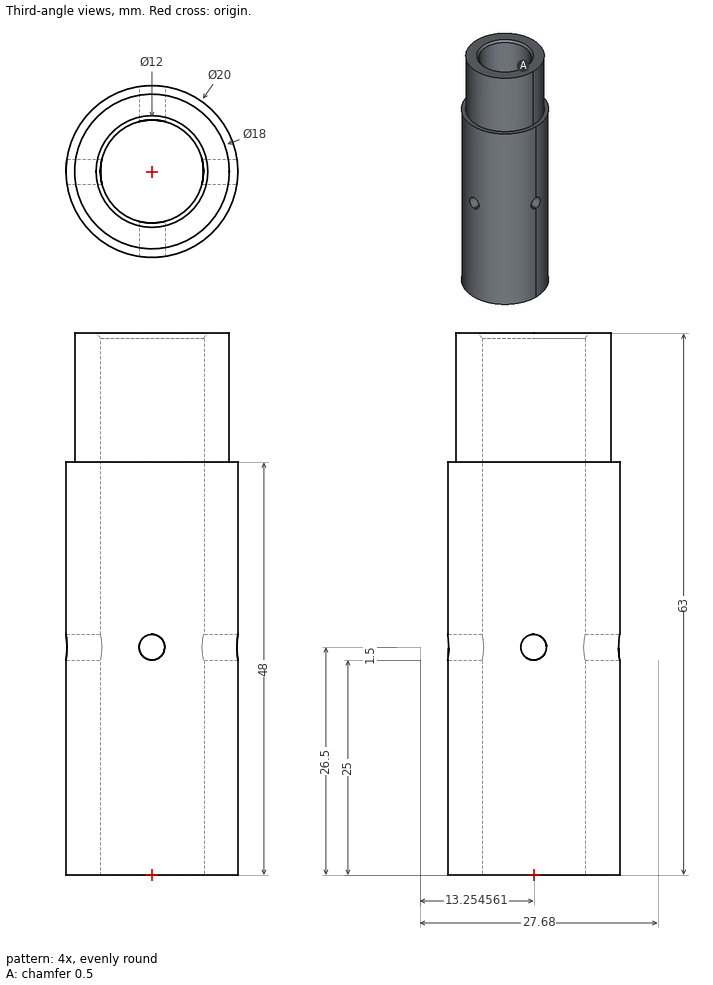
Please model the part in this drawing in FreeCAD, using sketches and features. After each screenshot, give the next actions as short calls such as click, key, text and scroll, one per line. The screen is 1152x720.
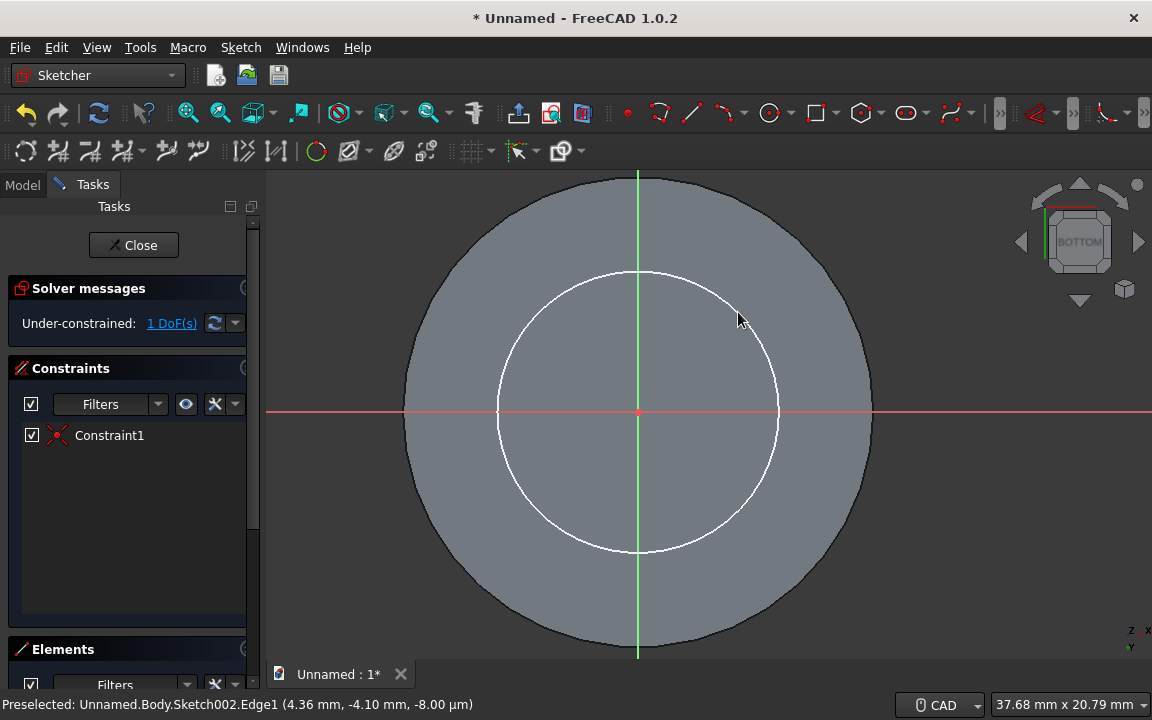
click(1036, 114)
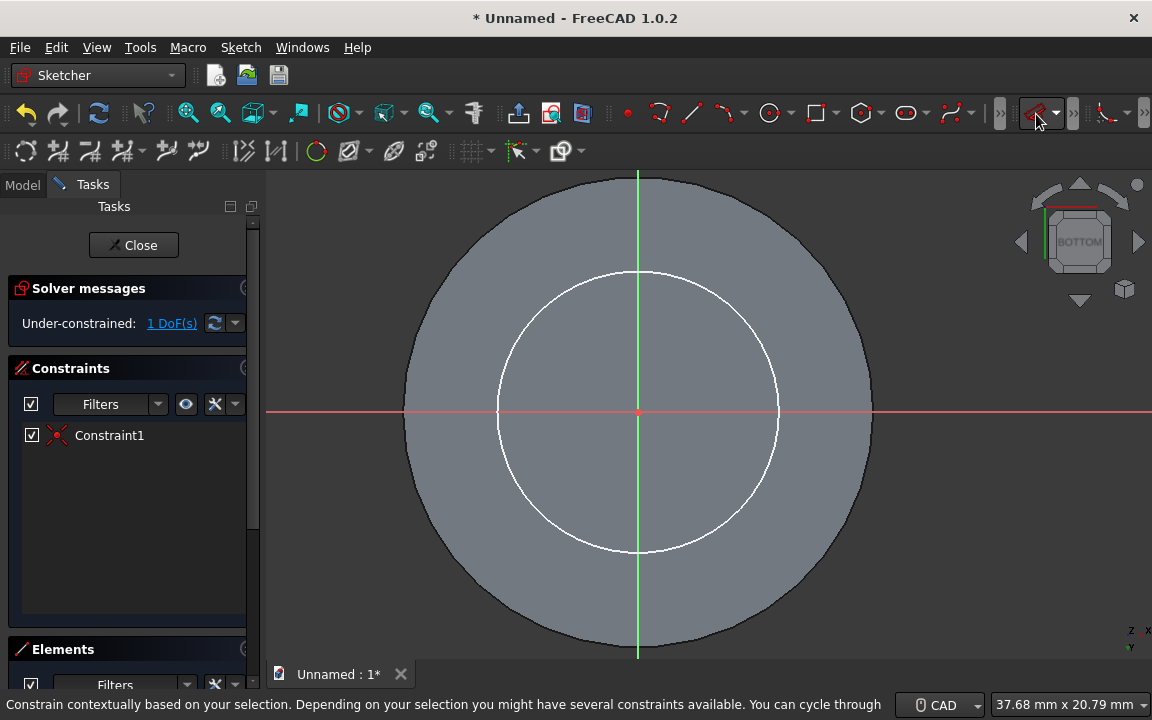
click(737, 312)
click(759, 289)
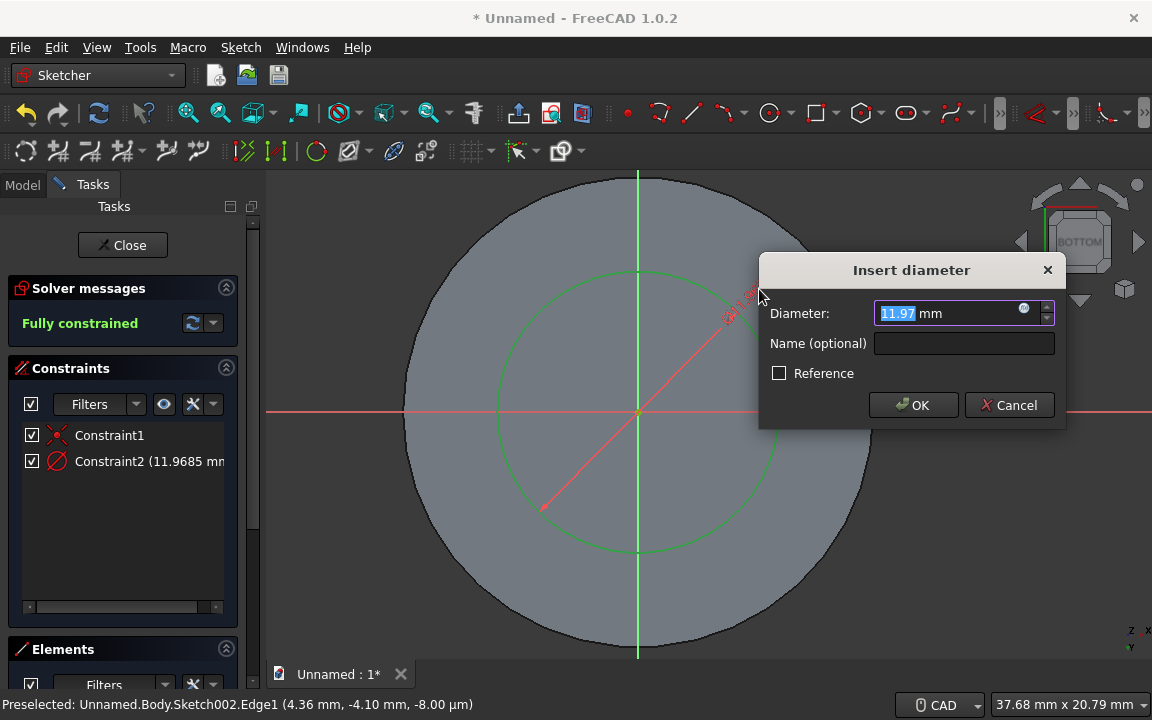
text(12)
key(Return)
key(Escape)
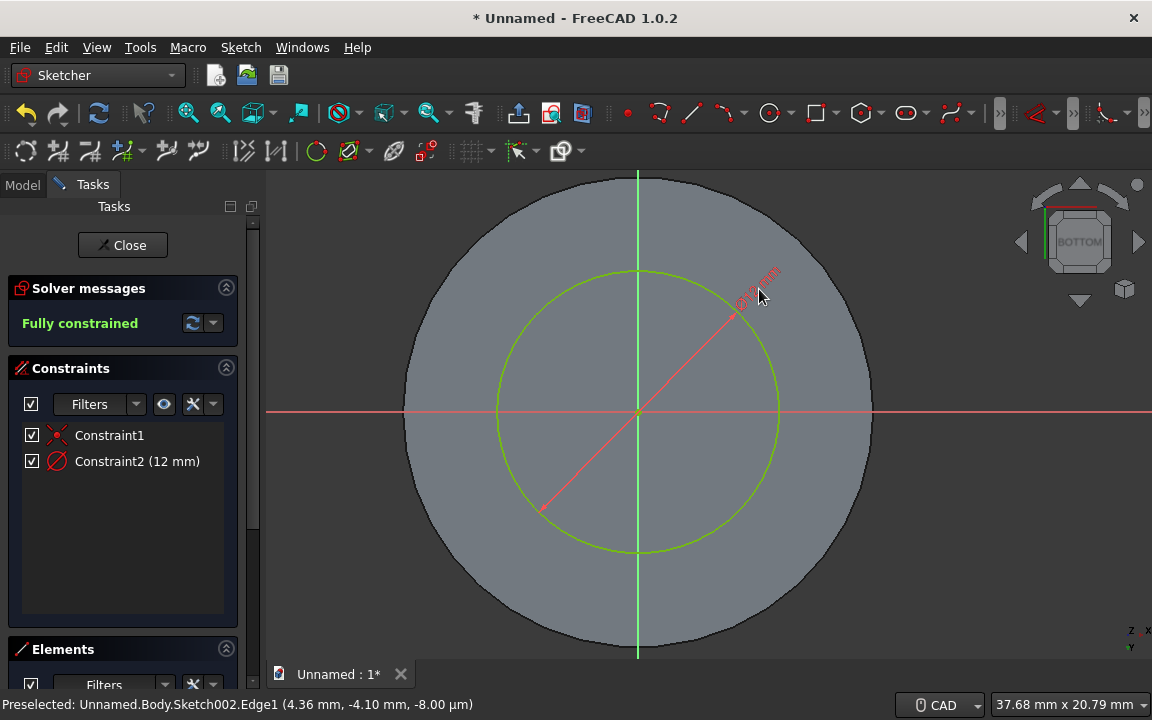
click(123, 245)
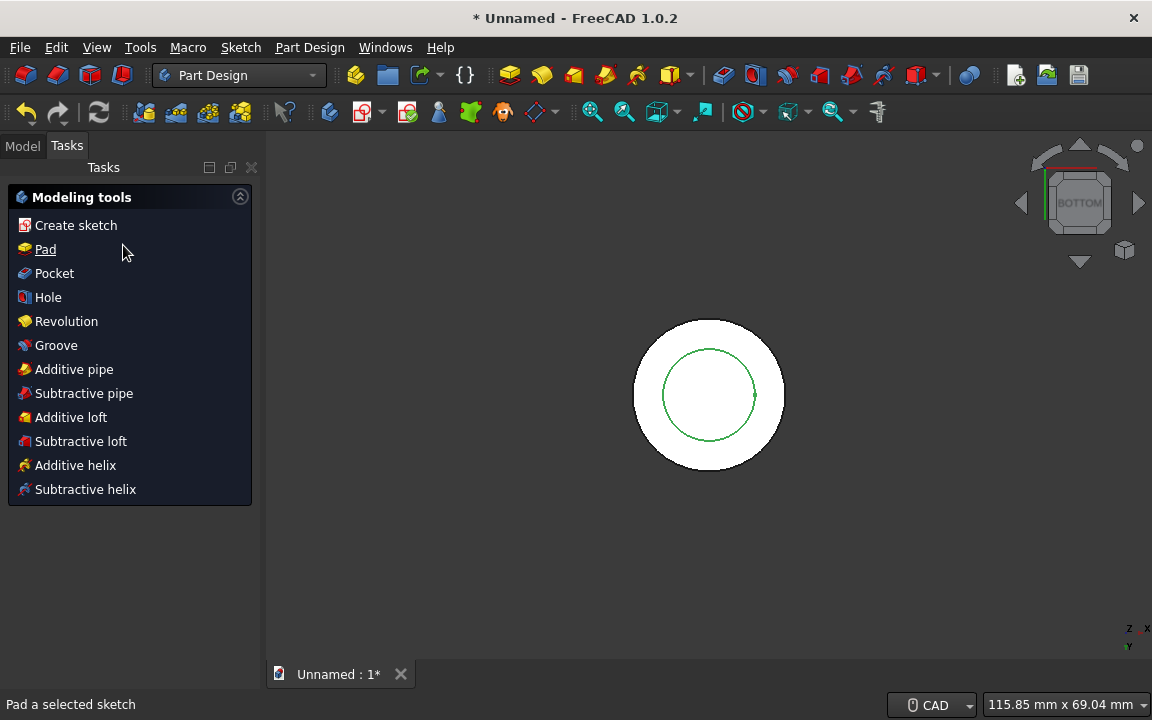
click(724, 76)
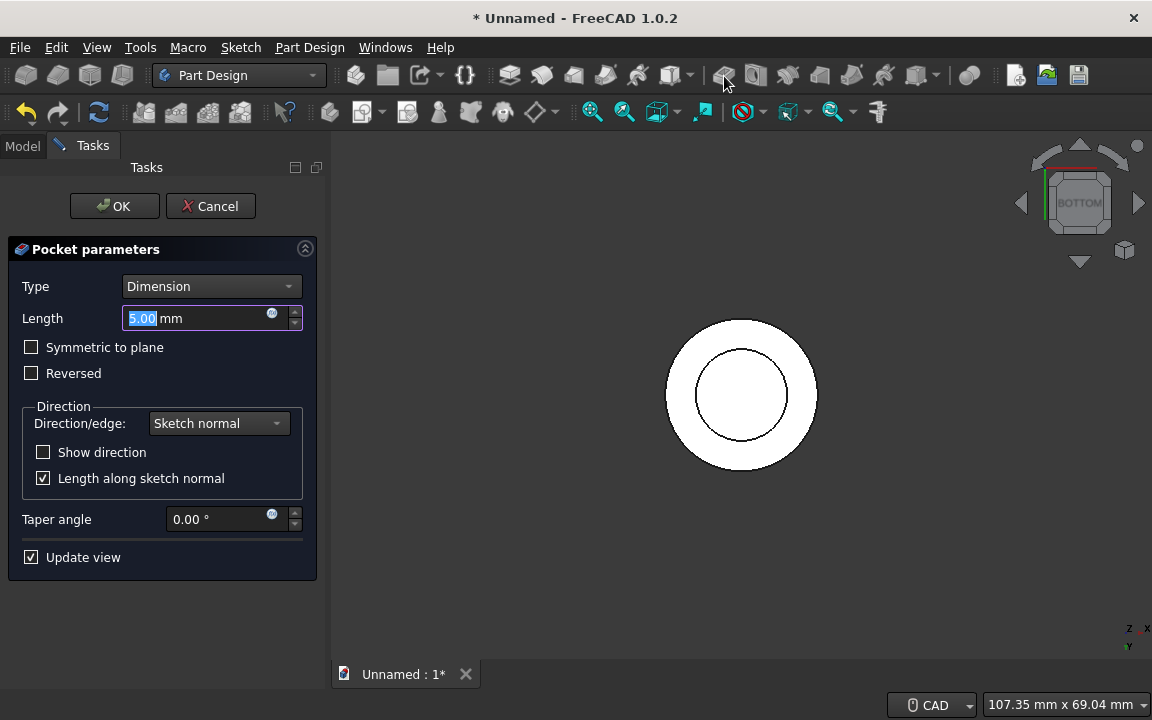
click(212, 286)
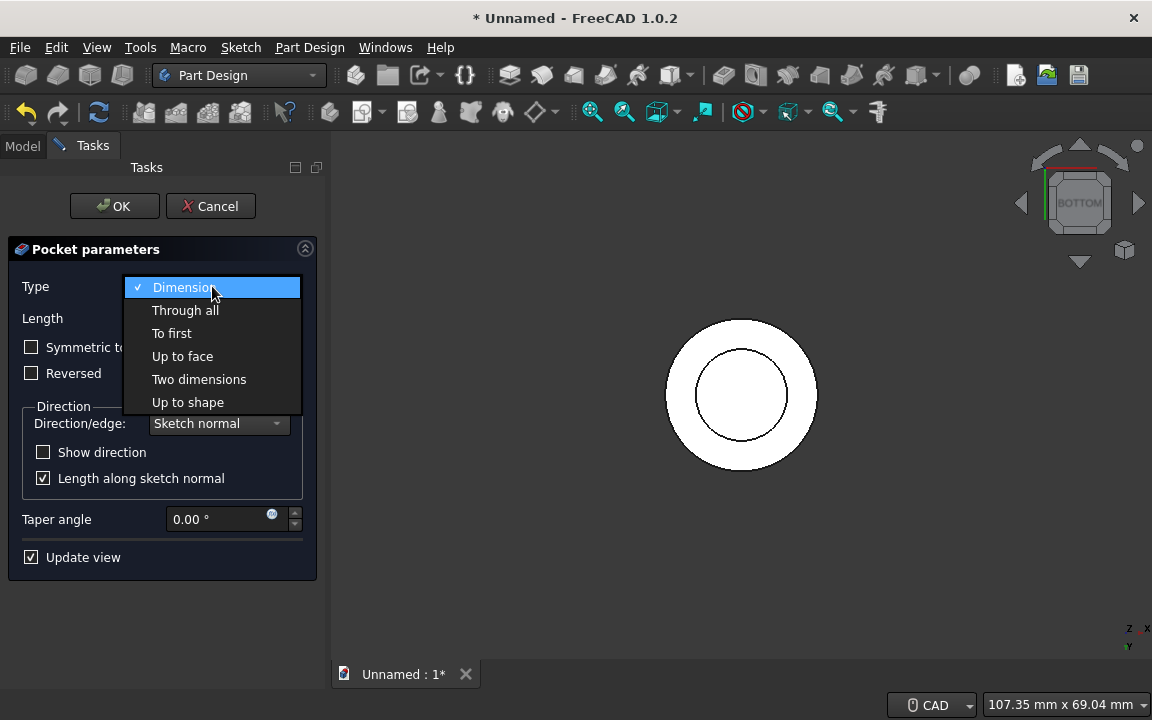
click(212, 310)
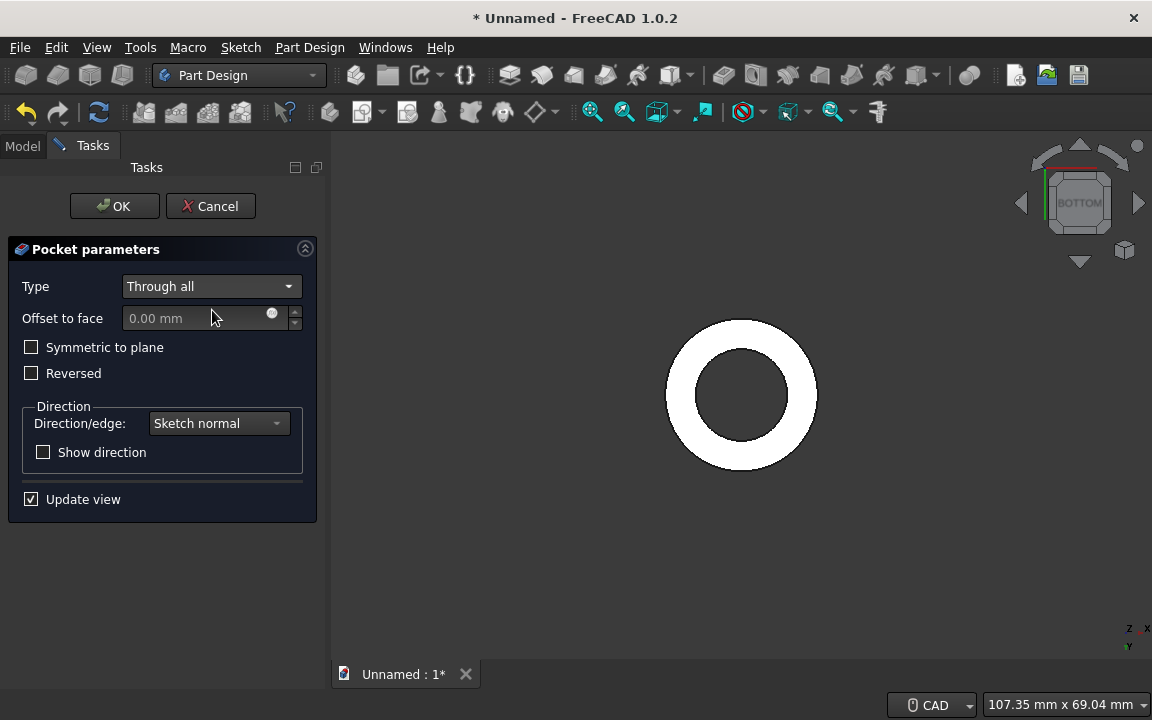
click(115, 206)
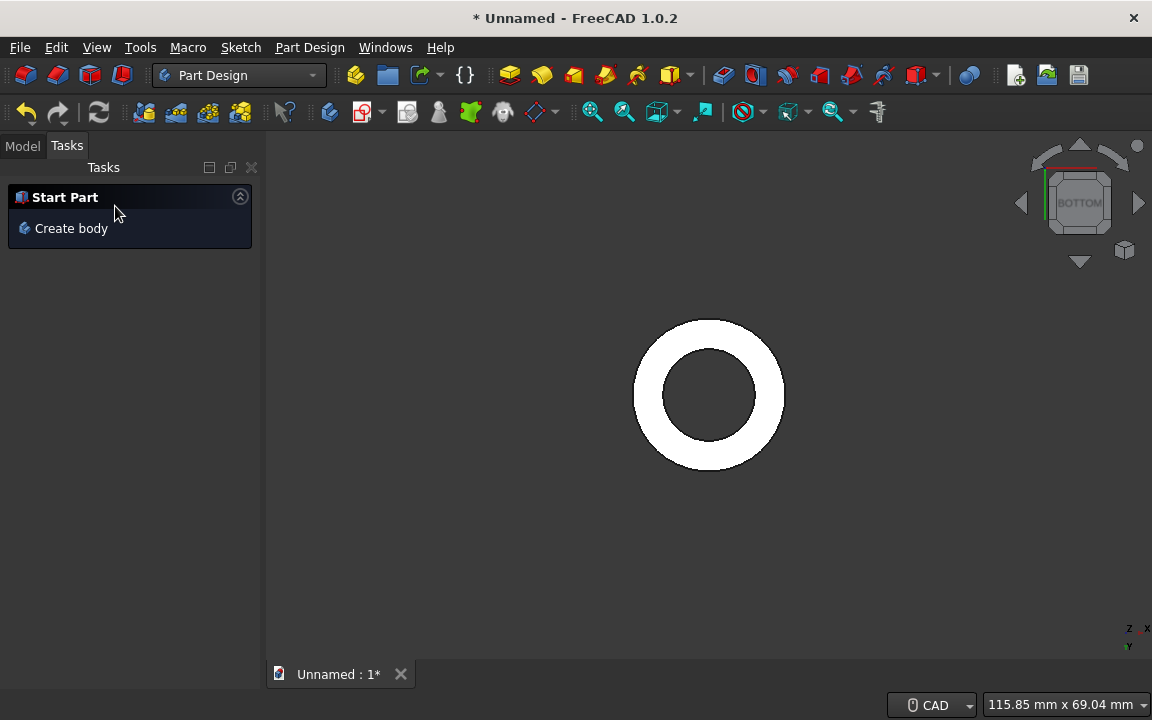
click(594, 112)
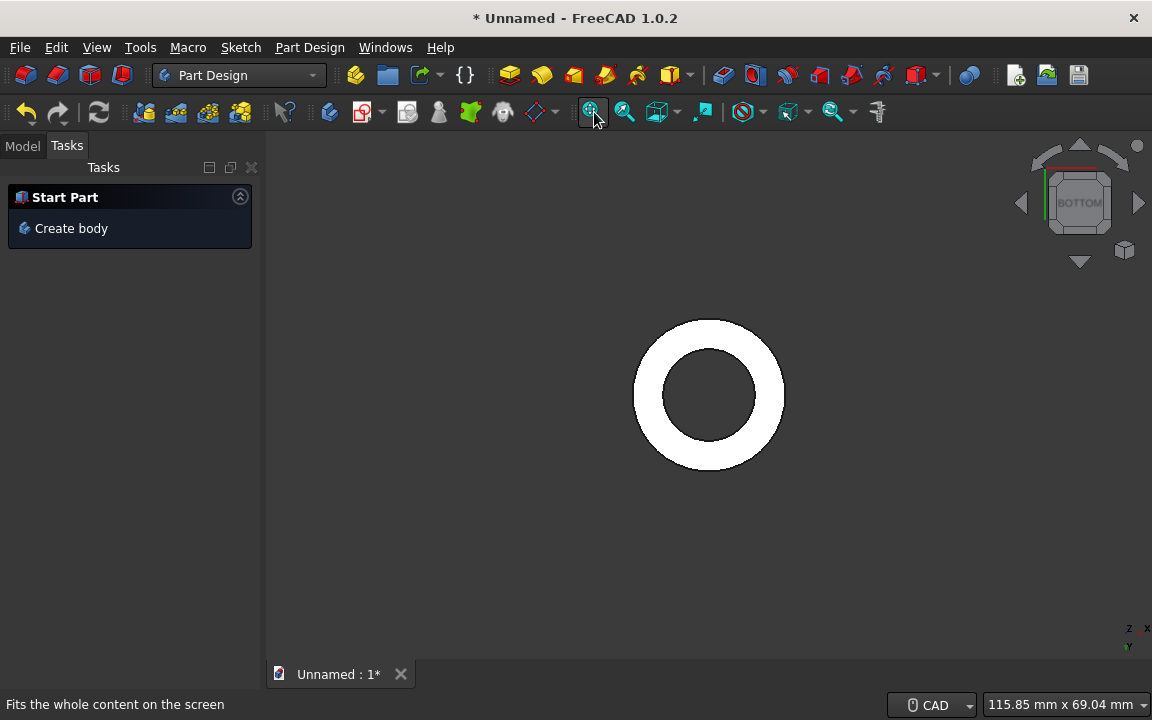
click(362, 112)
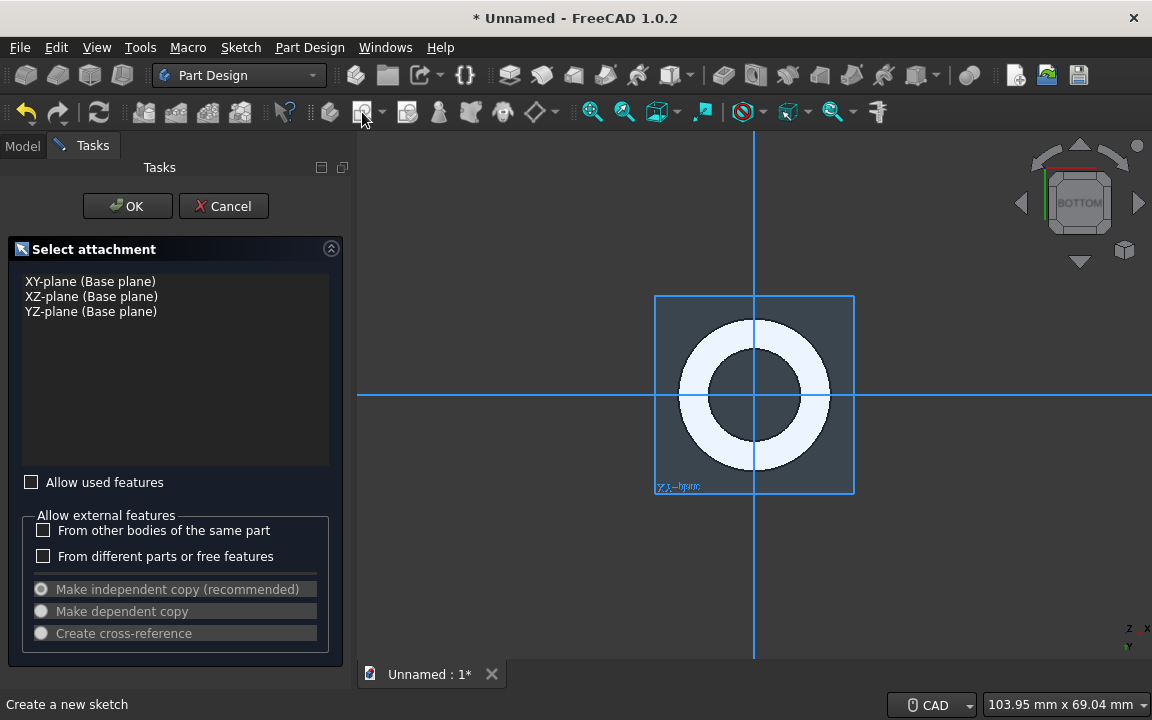
click(82, 312)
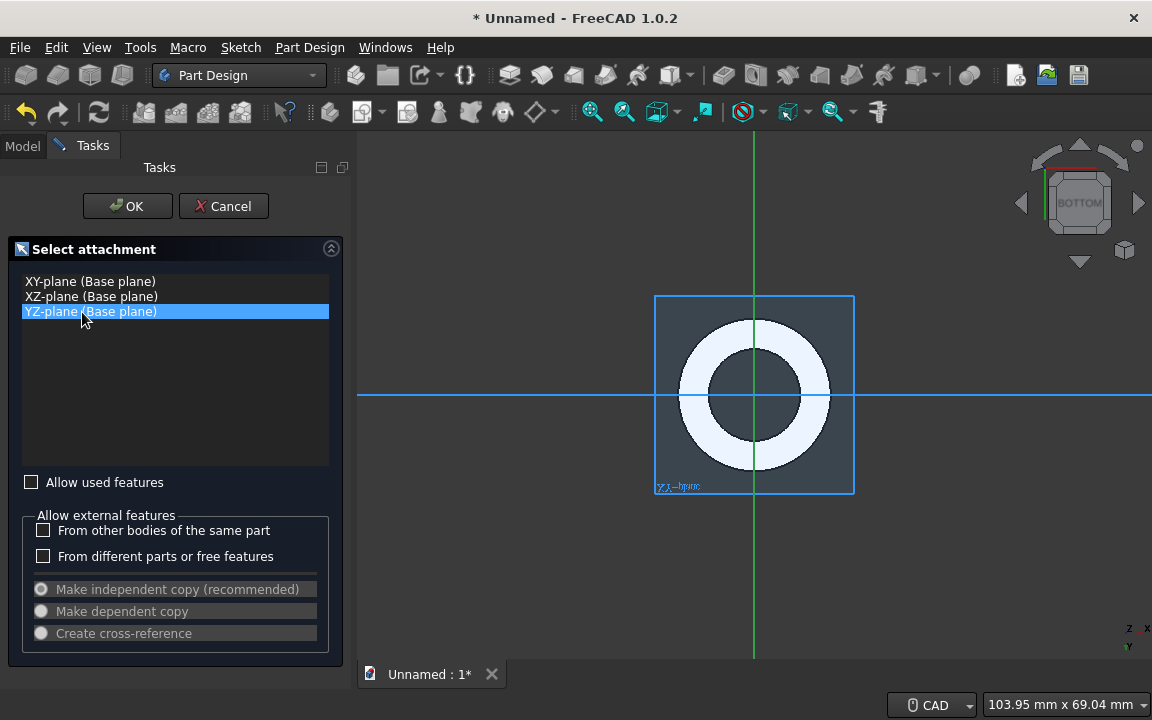
click(128, 206)